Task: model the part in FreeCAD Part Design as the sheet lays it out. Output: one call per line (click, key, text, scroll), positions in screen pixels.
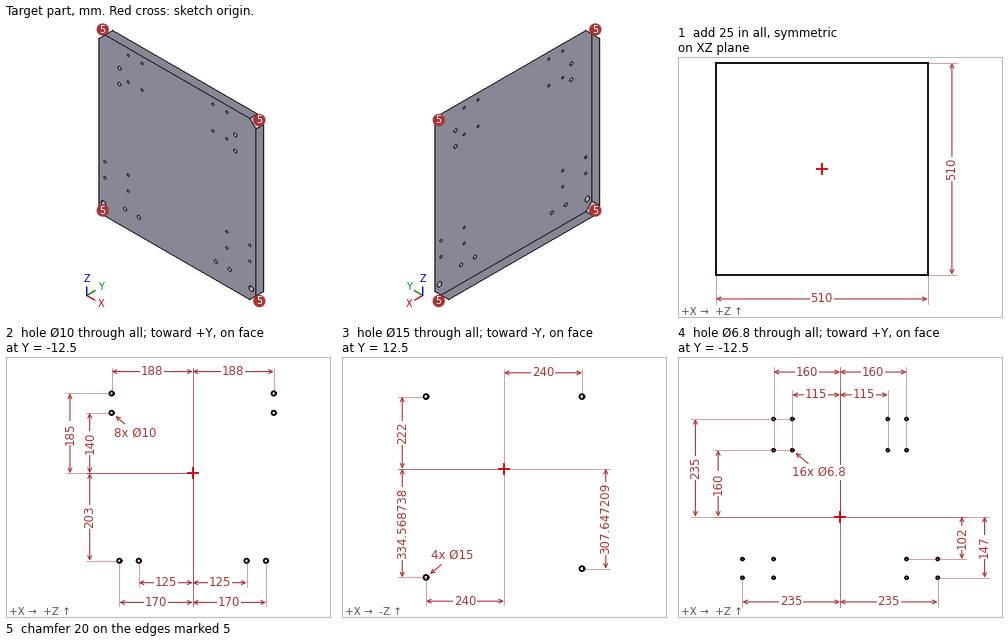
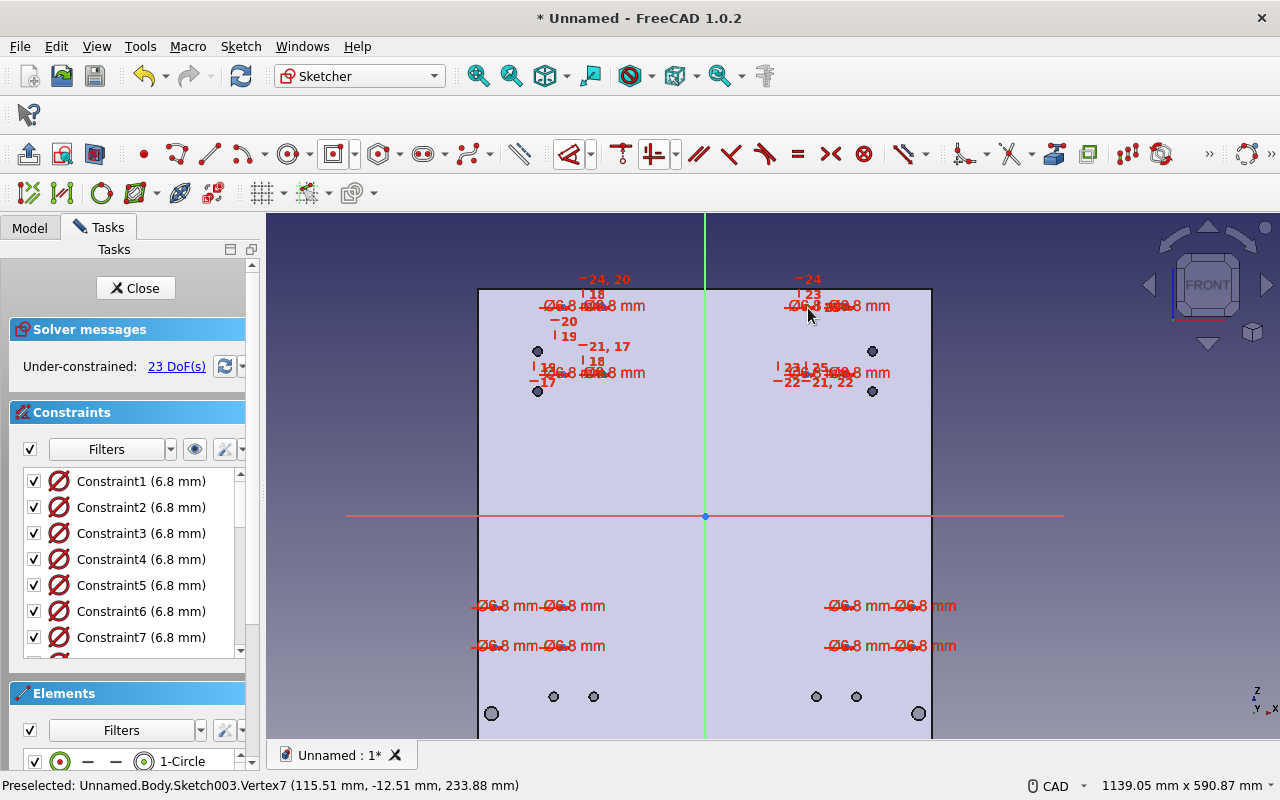
click(848, 308)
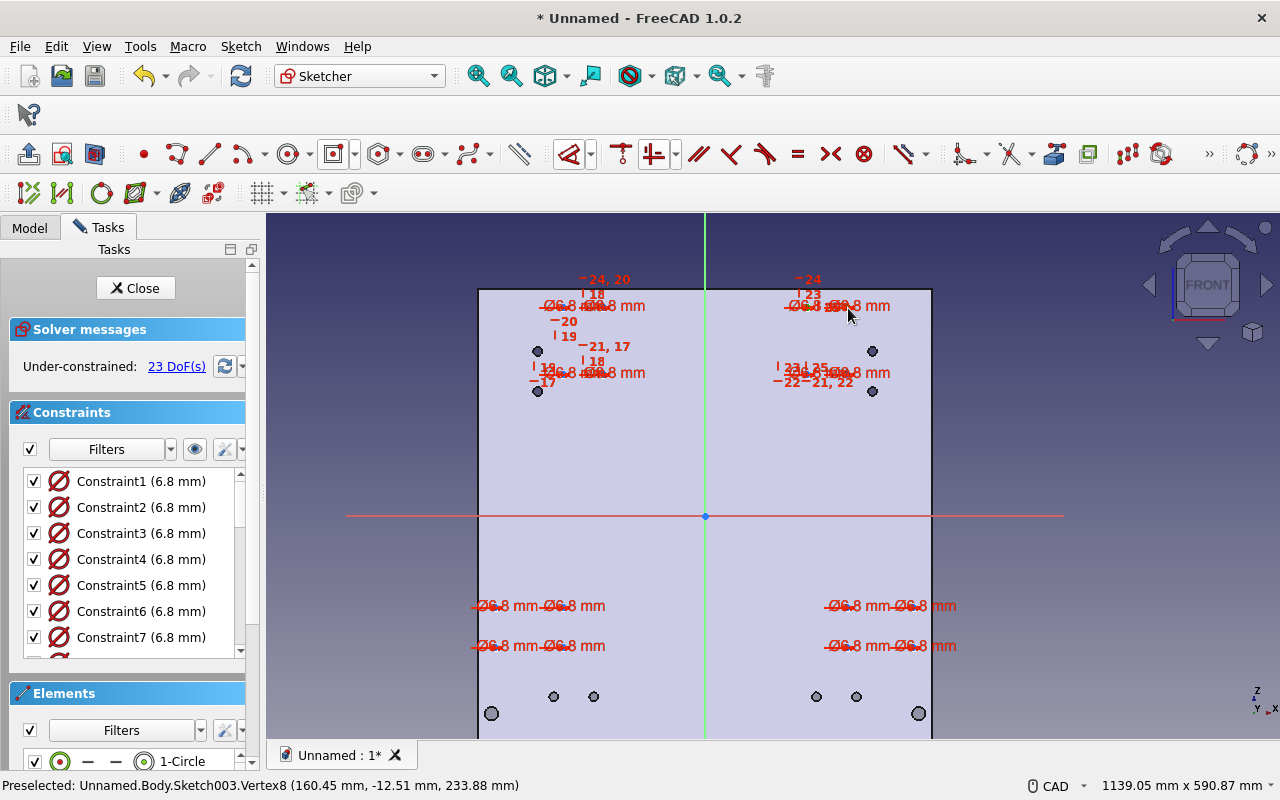
key(h)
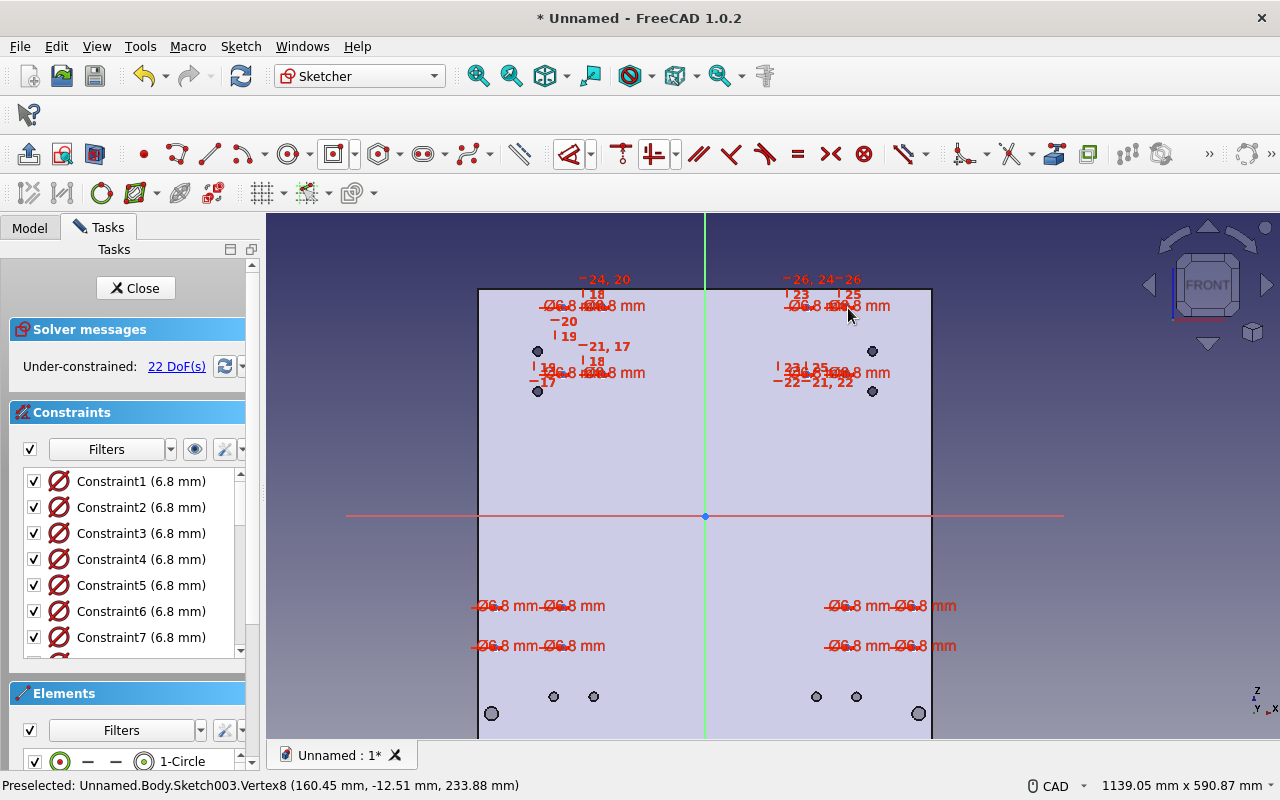
click(848, 375)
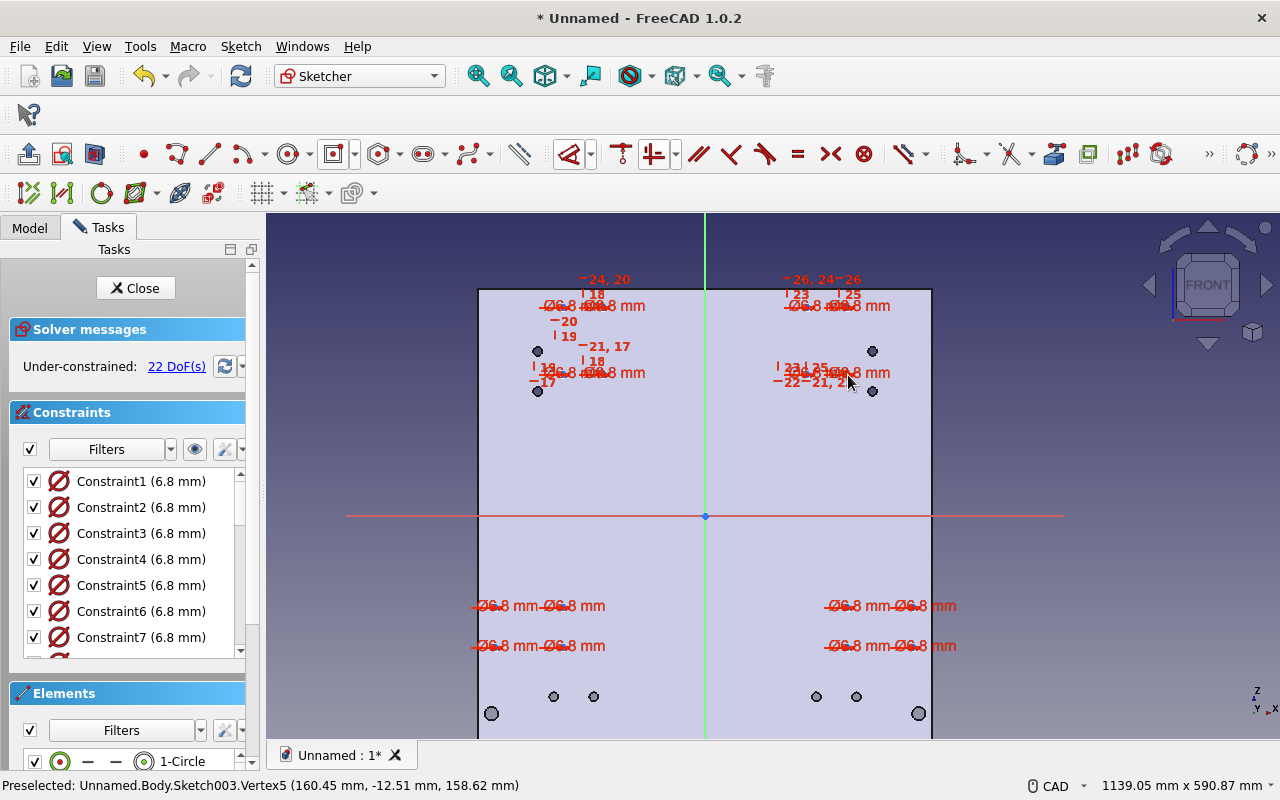
click(848, 648)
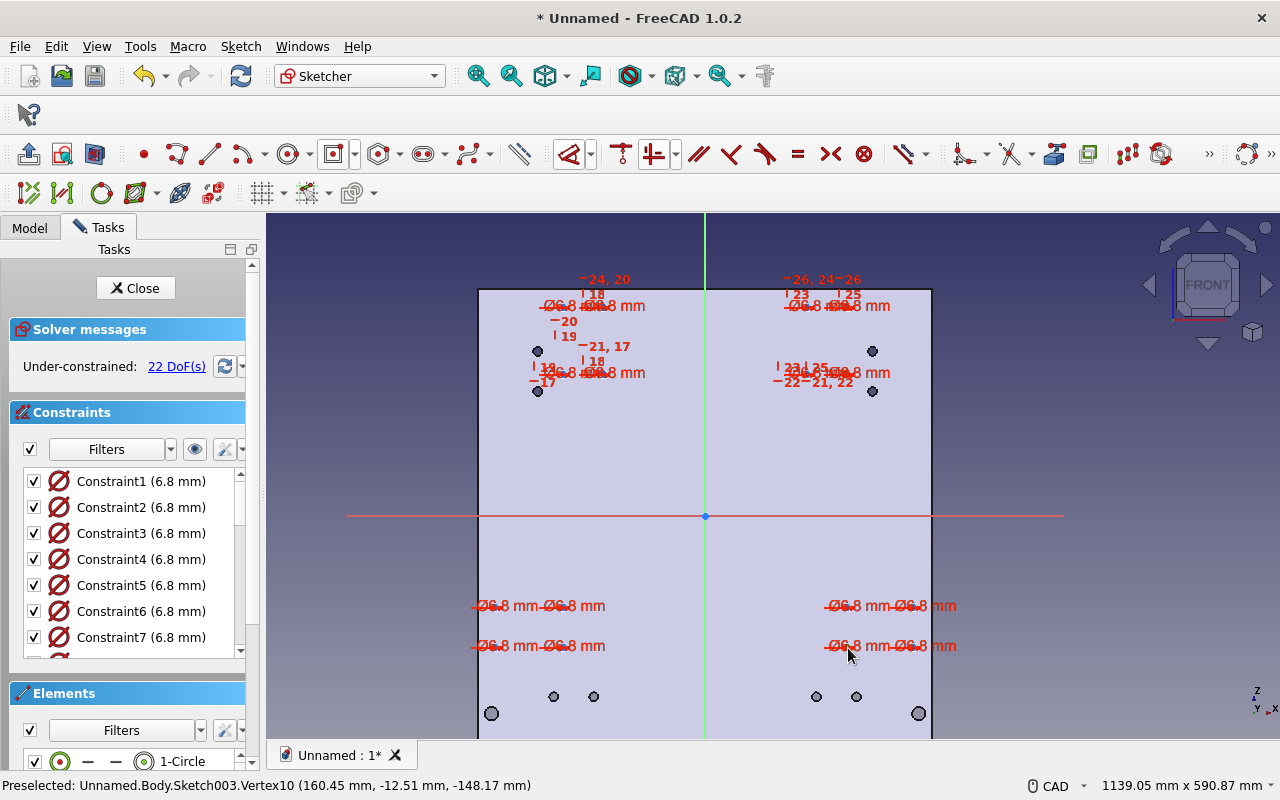
click(676, 154)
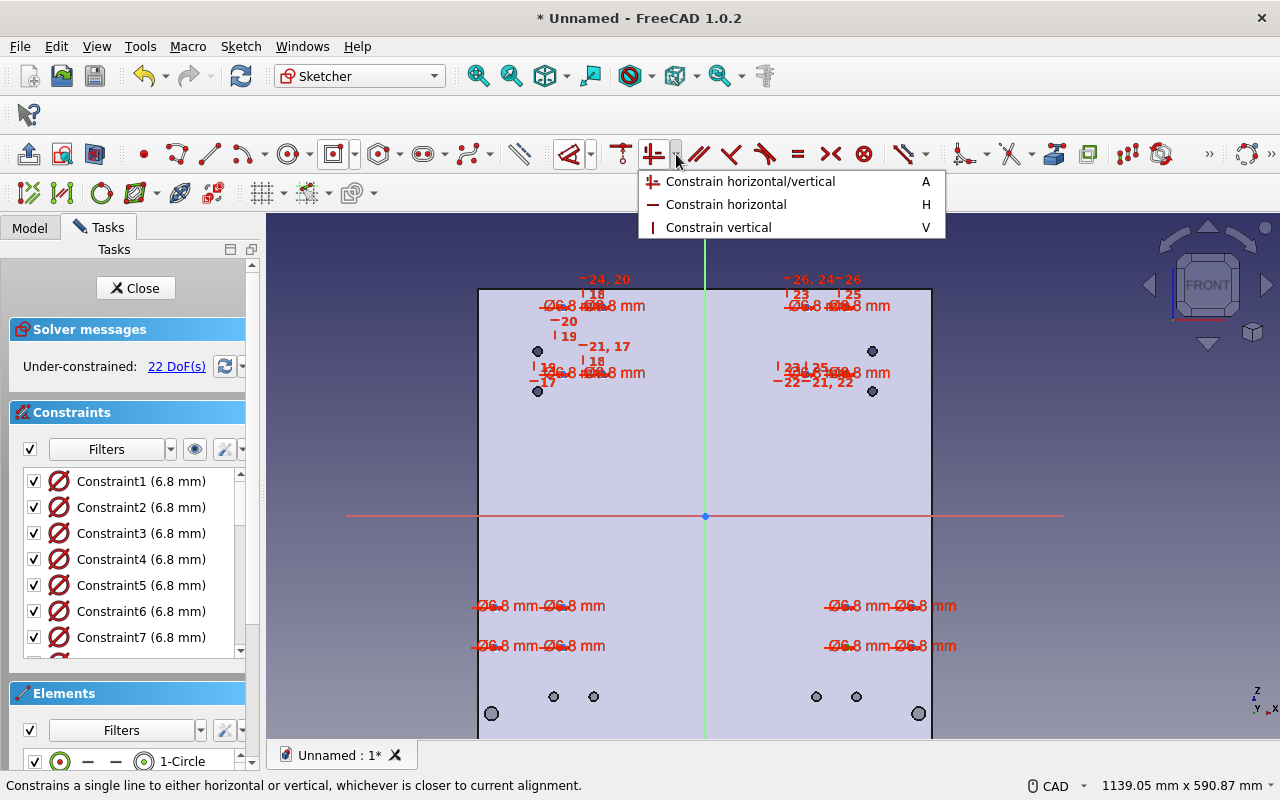
click(792, 228)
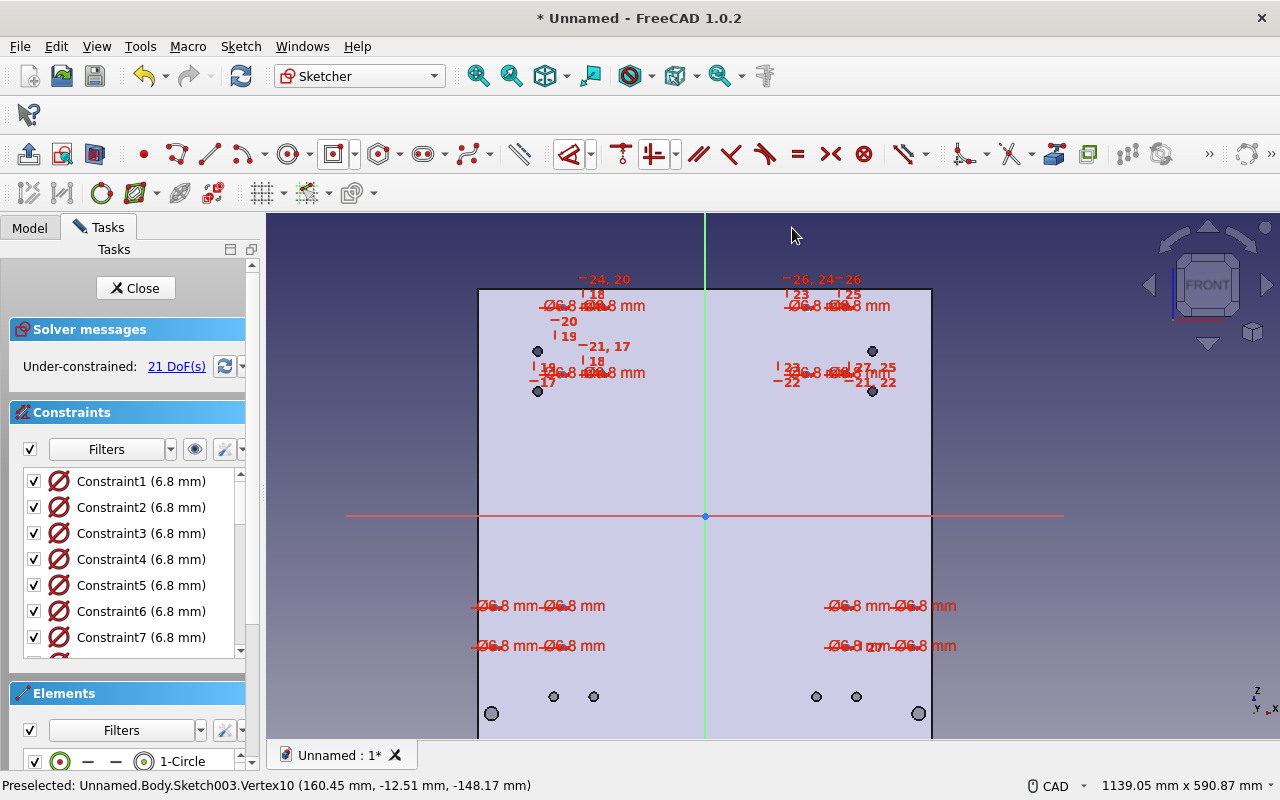
click(914, 648)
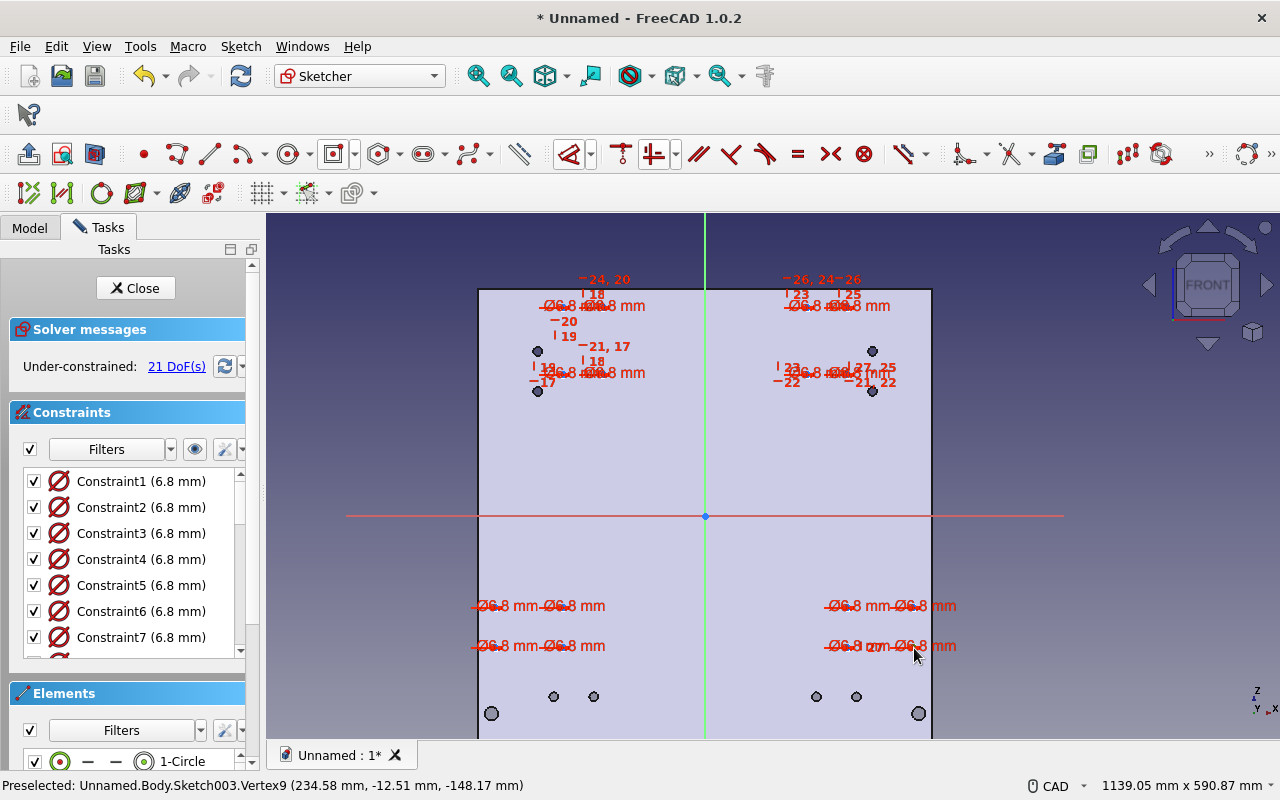
click(848, 648)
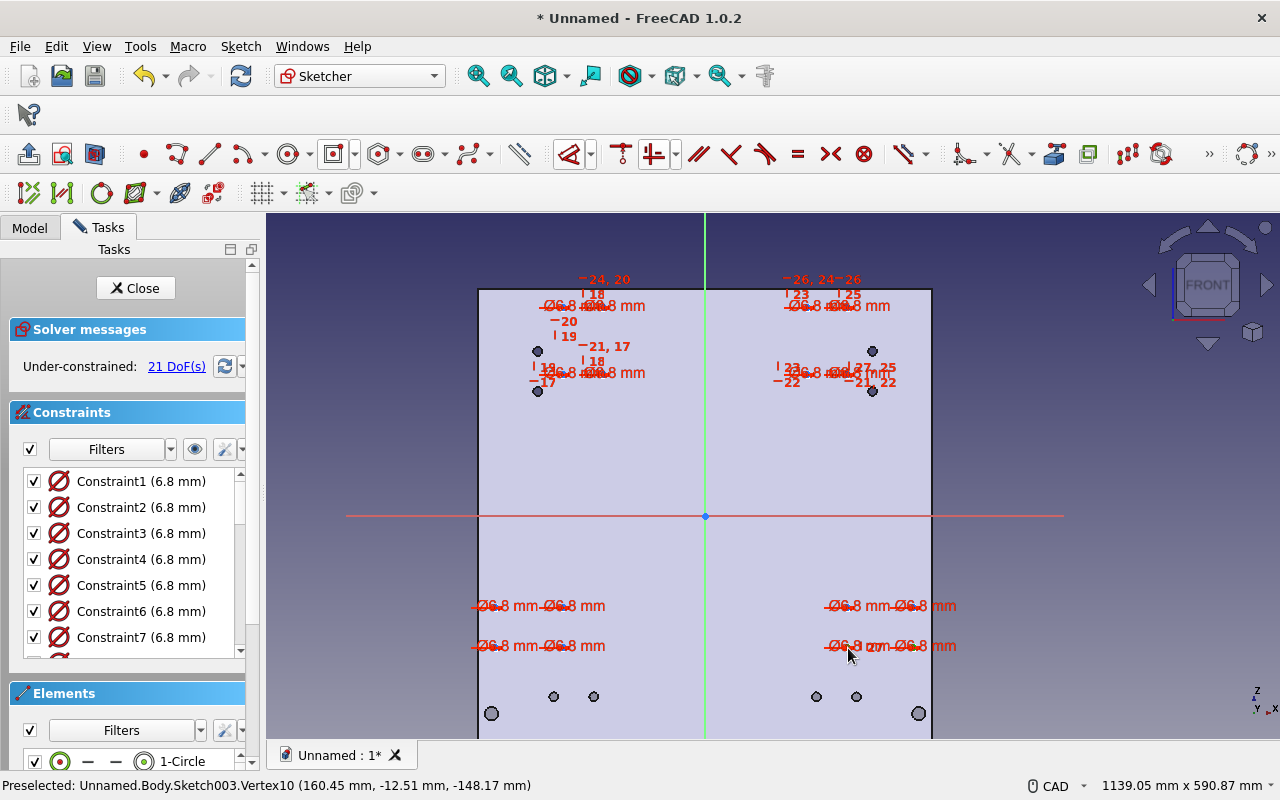
click(676, 154)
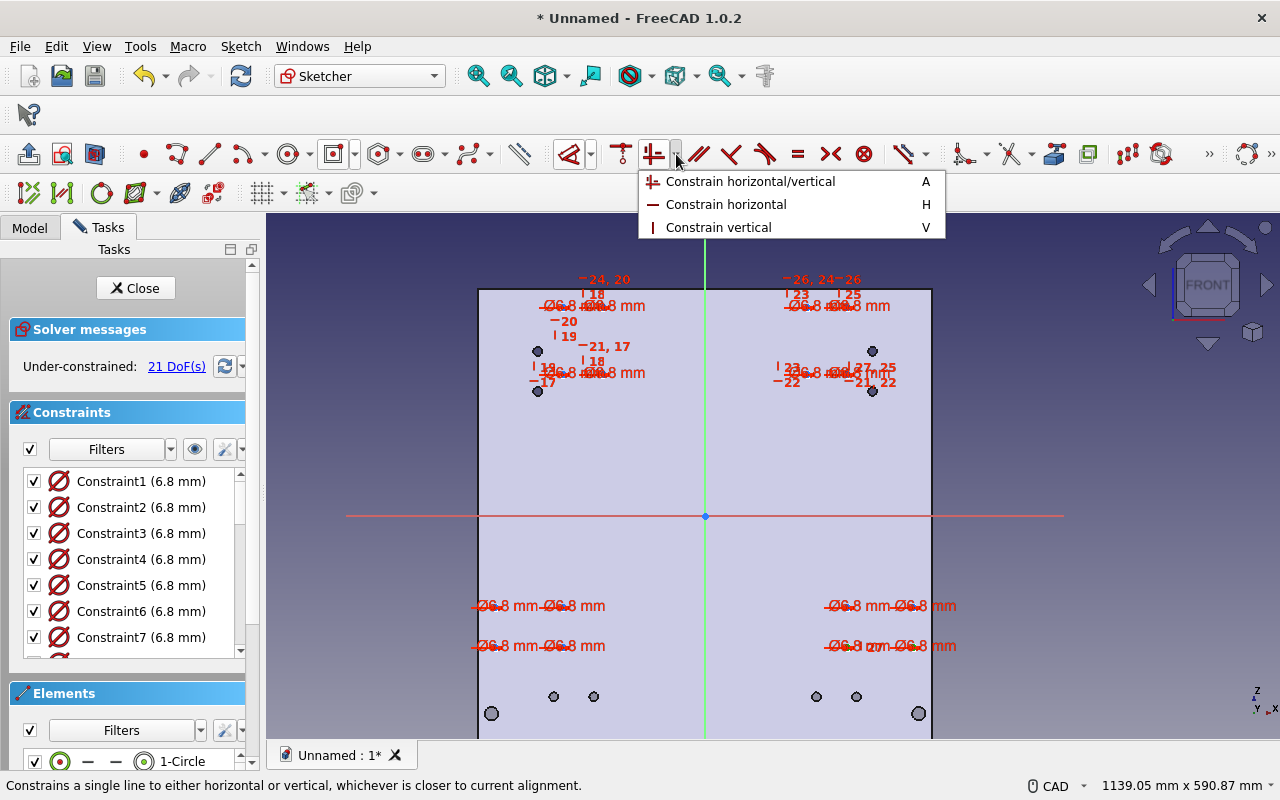
click(792, 204)